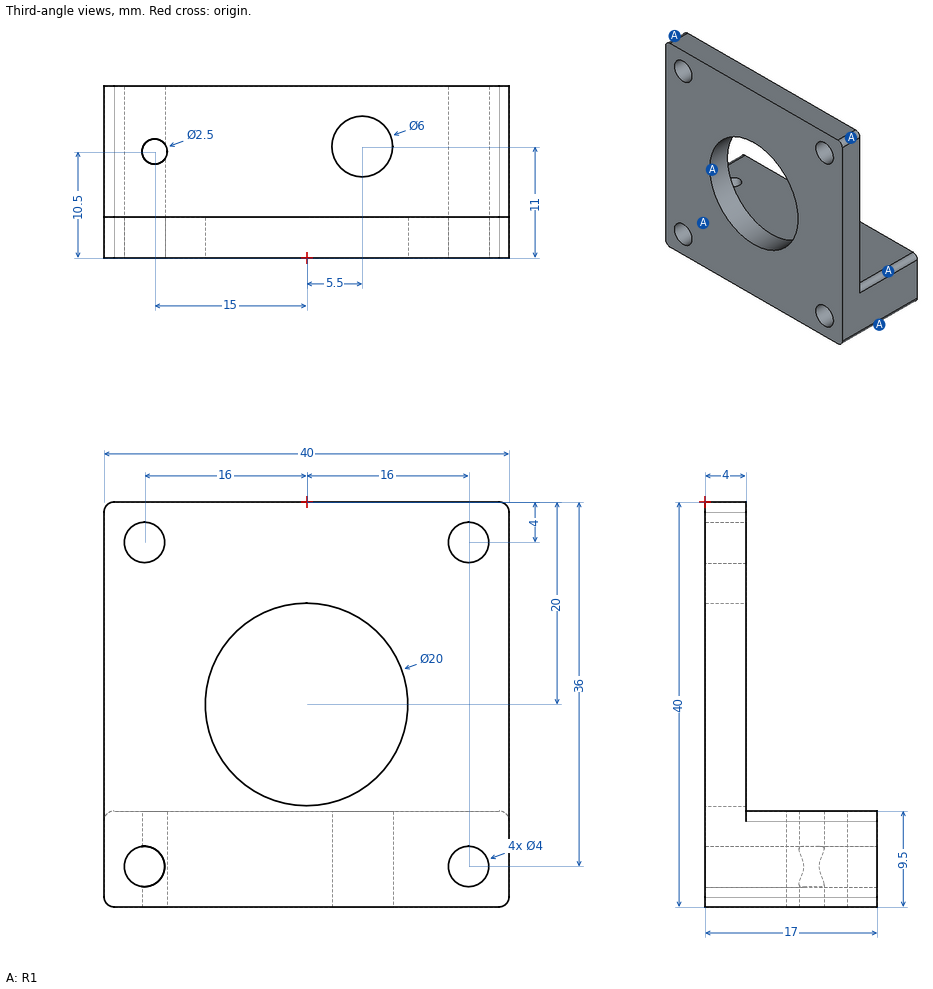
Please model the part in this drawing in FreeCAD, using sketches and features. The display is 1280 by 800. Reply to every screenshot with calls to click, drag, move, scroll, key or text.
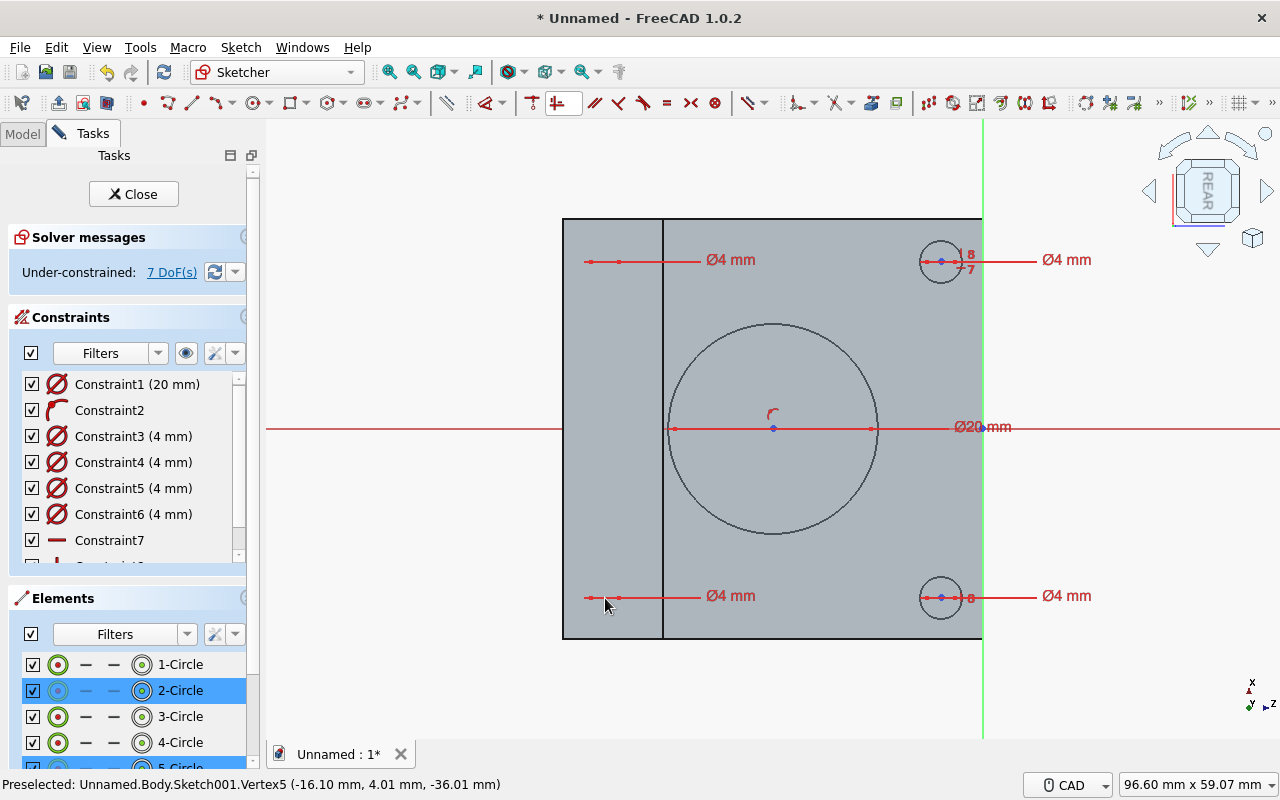
key(v)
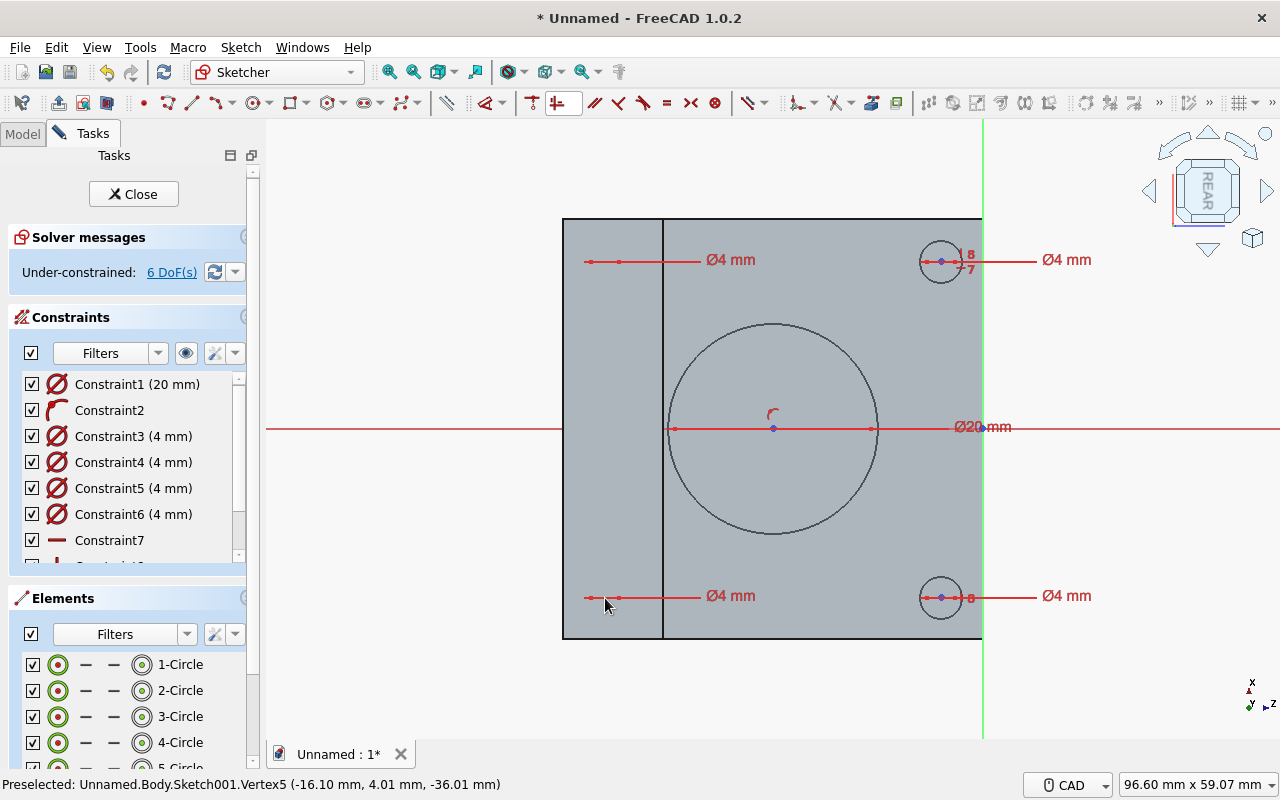
click(941, 598)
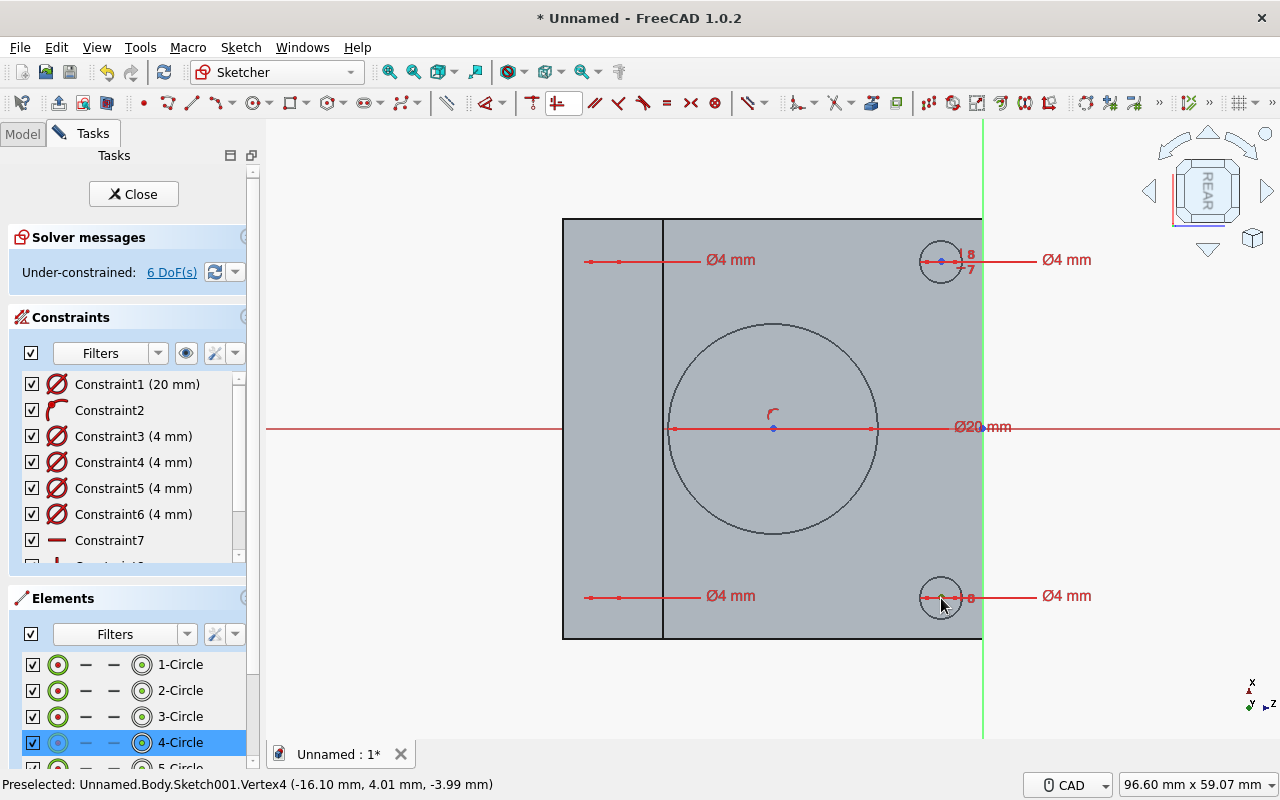
click(605, 598)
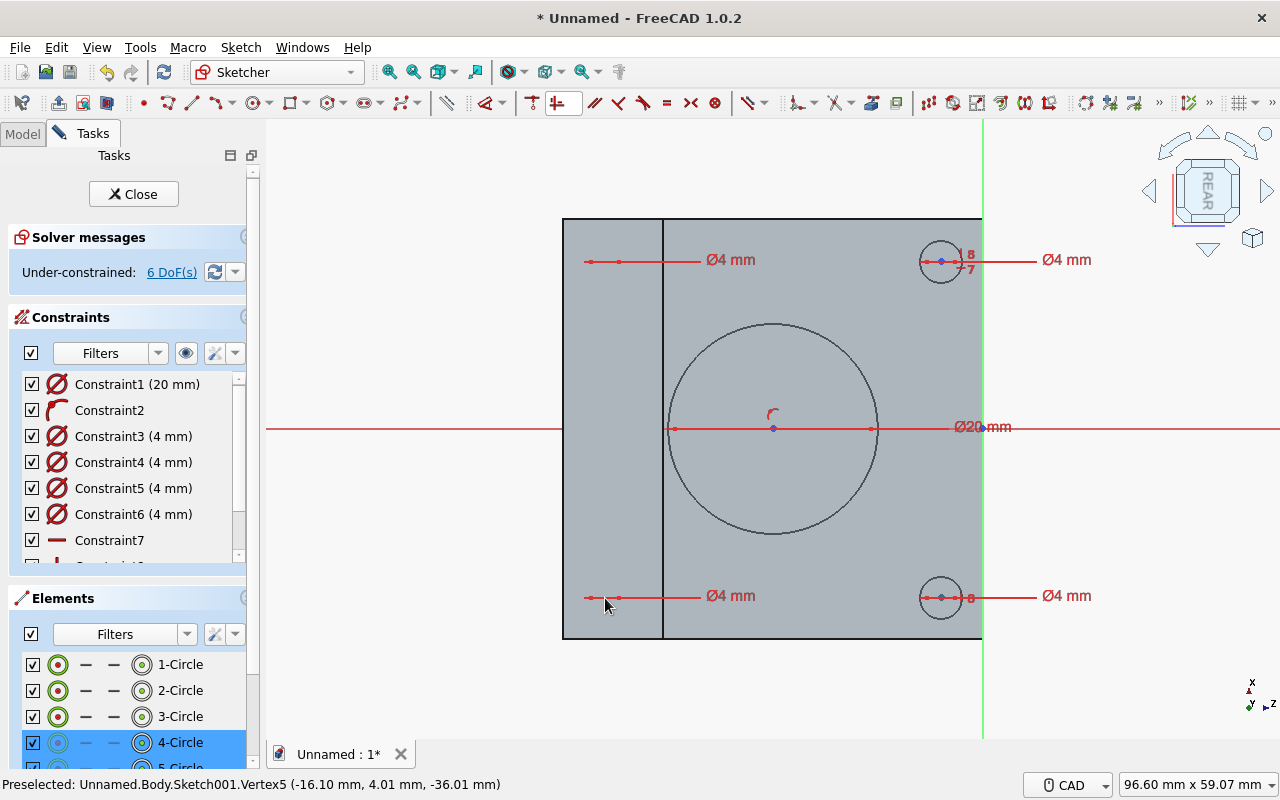
key(h)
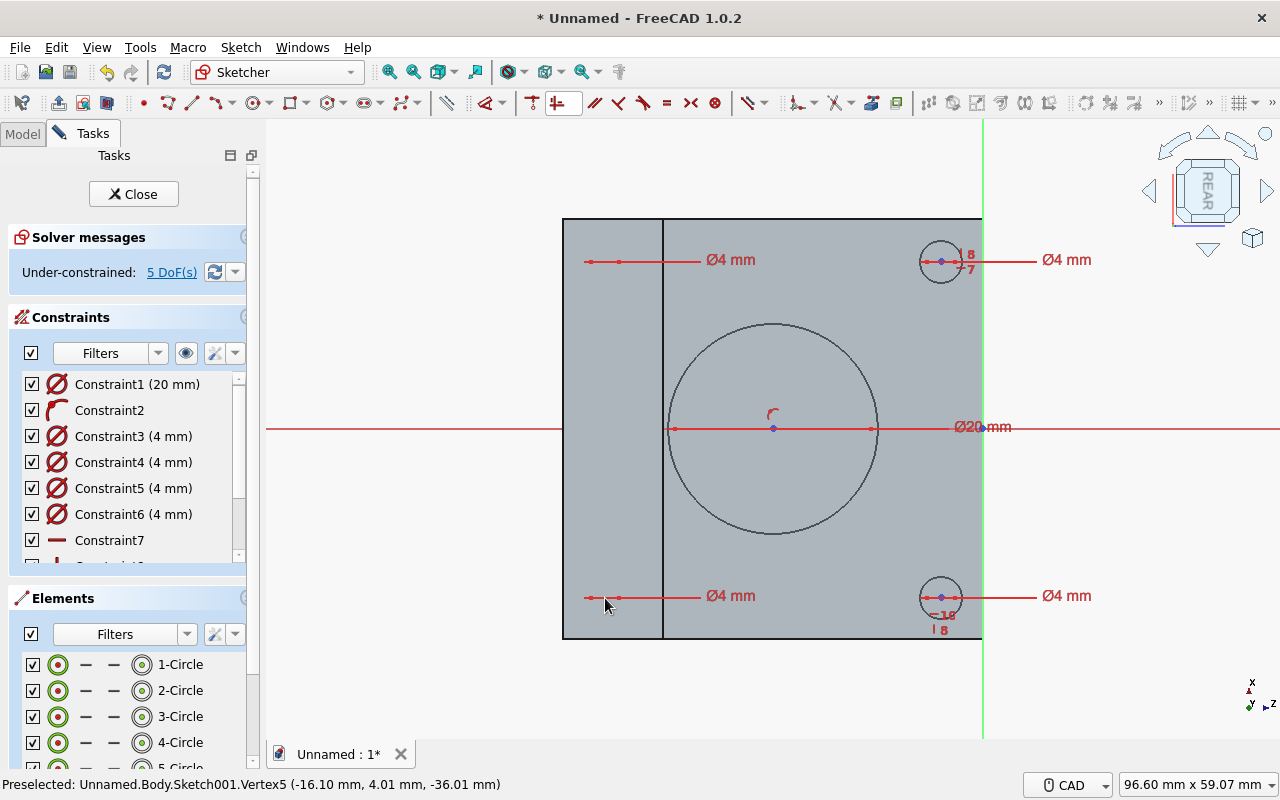
key(d)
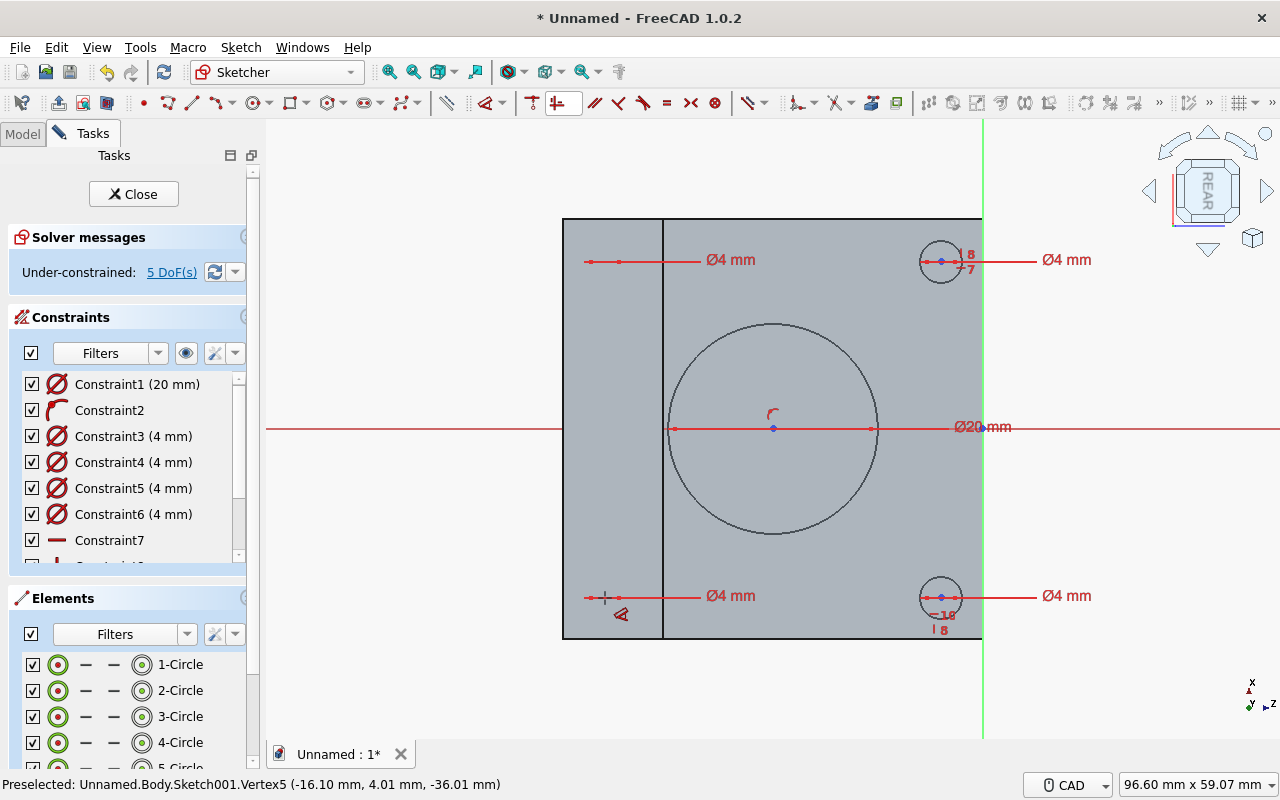
click(941, 262)
click(962, 228)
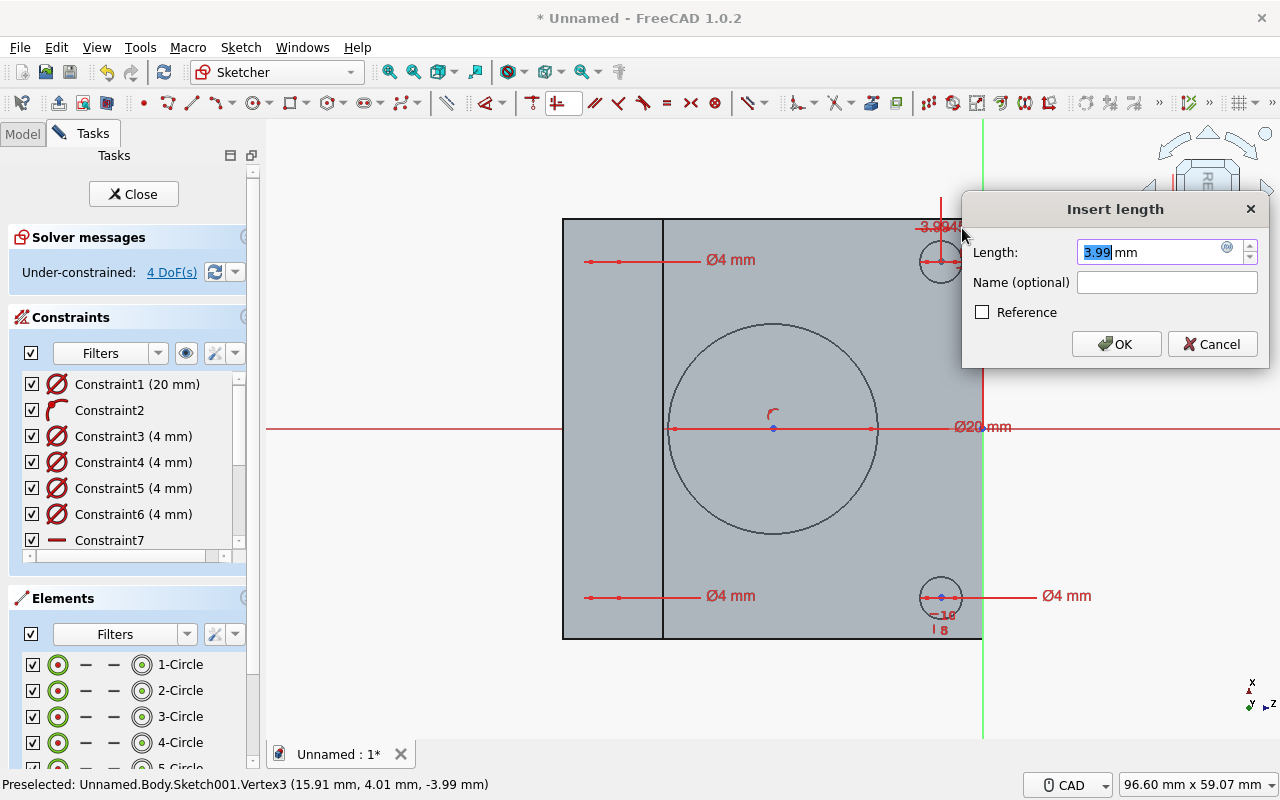
text(4)
key(Return)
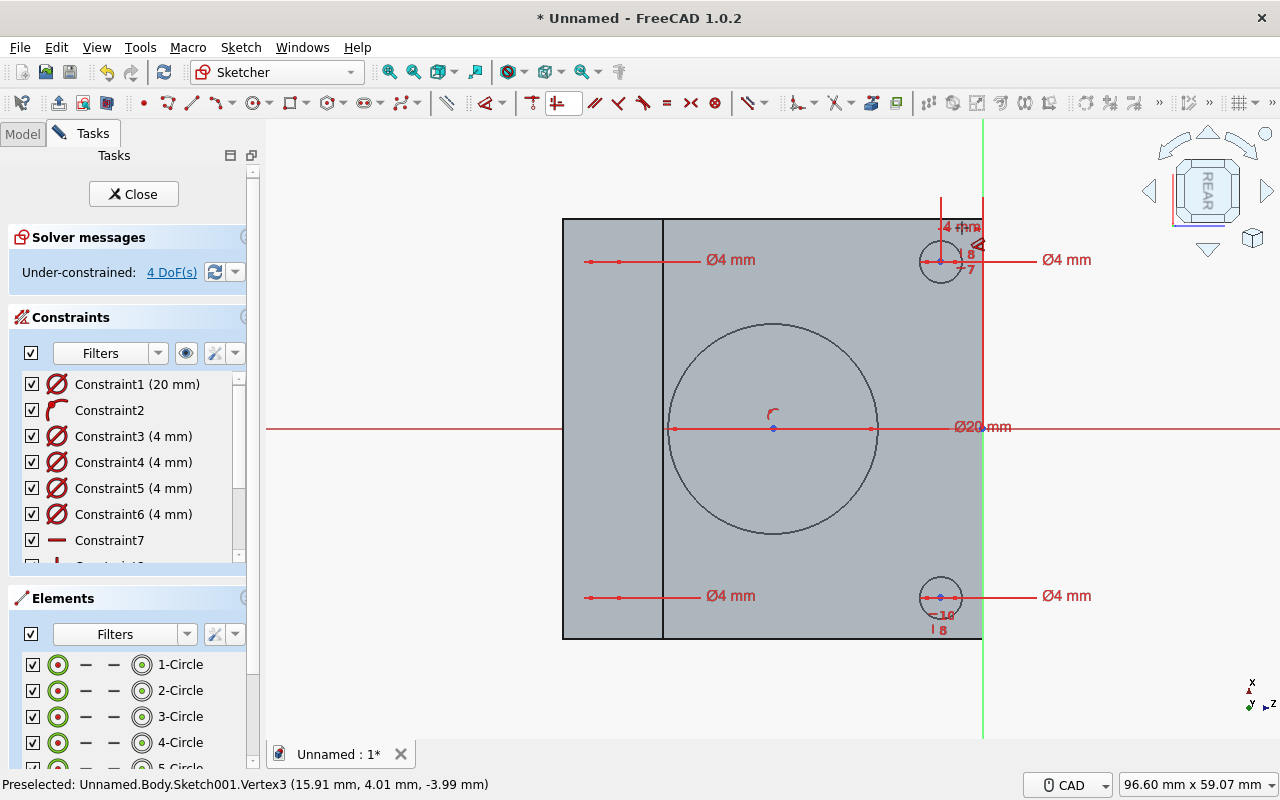
click(773, 429)
click(830, 463)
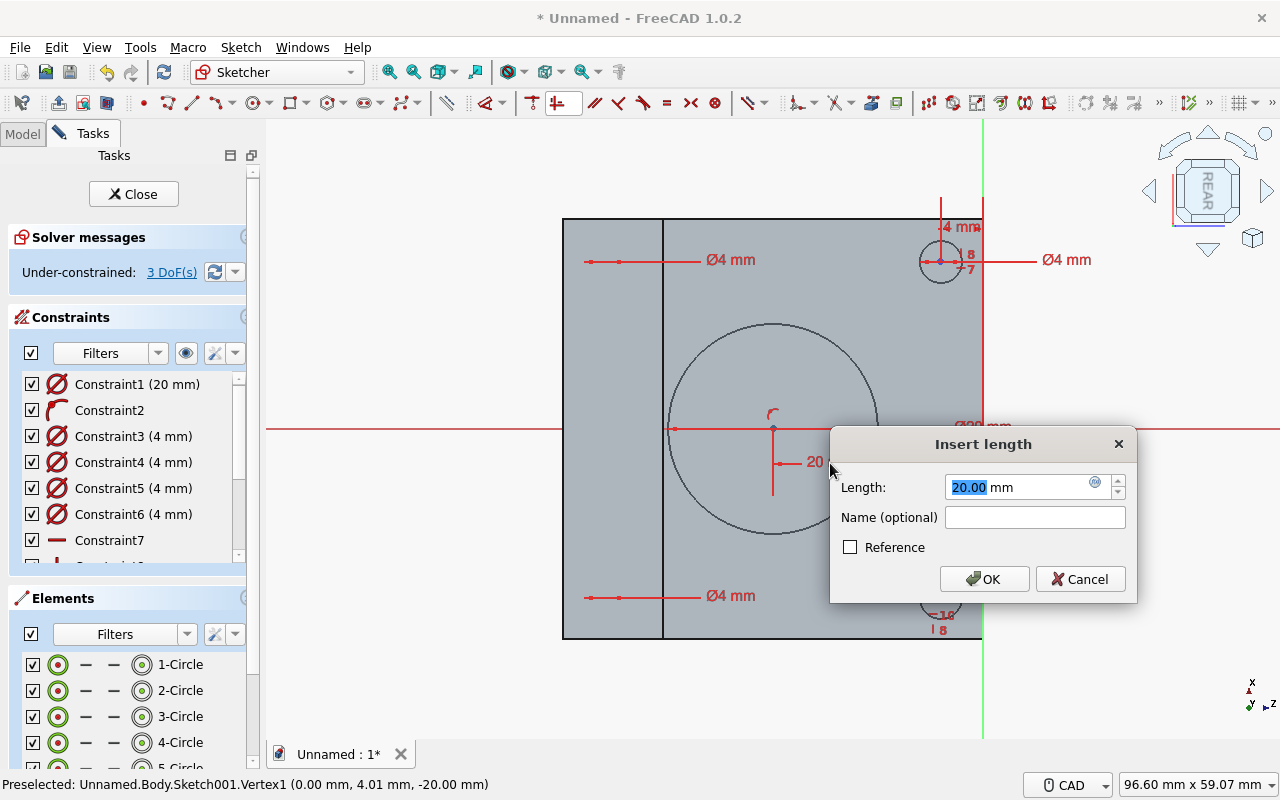
text(20)
key(Return)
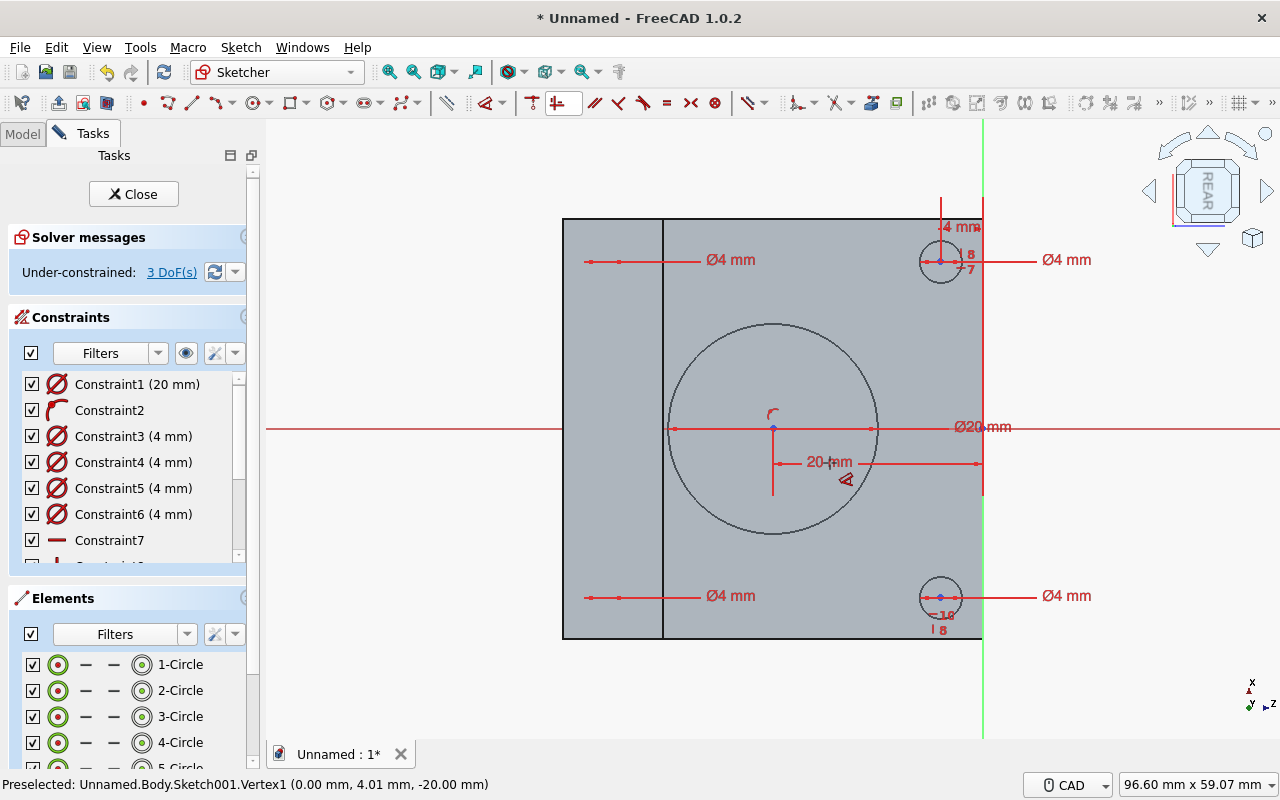
click(605, 262)
click(794, 228)